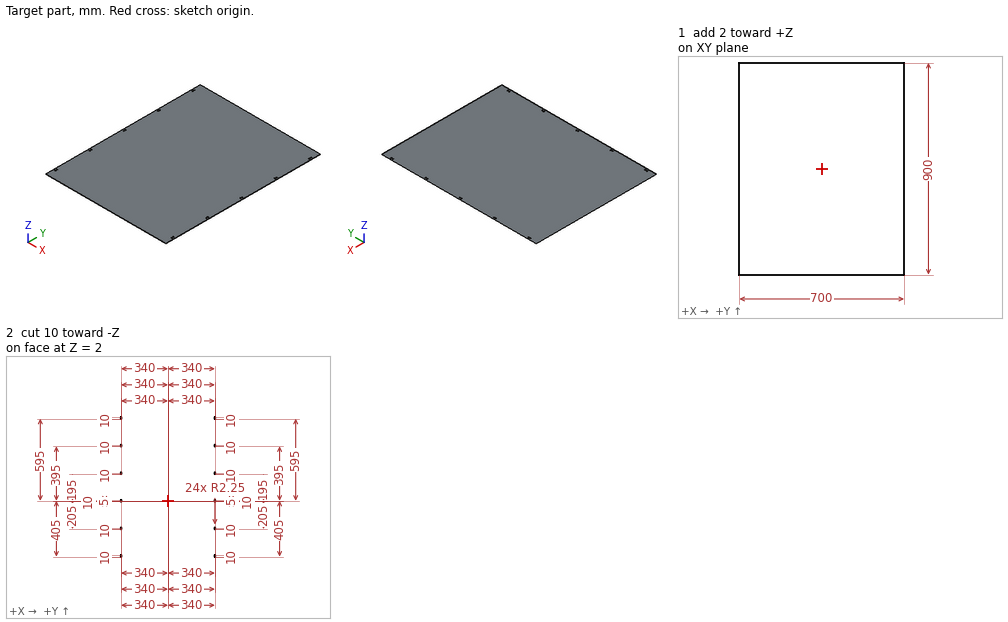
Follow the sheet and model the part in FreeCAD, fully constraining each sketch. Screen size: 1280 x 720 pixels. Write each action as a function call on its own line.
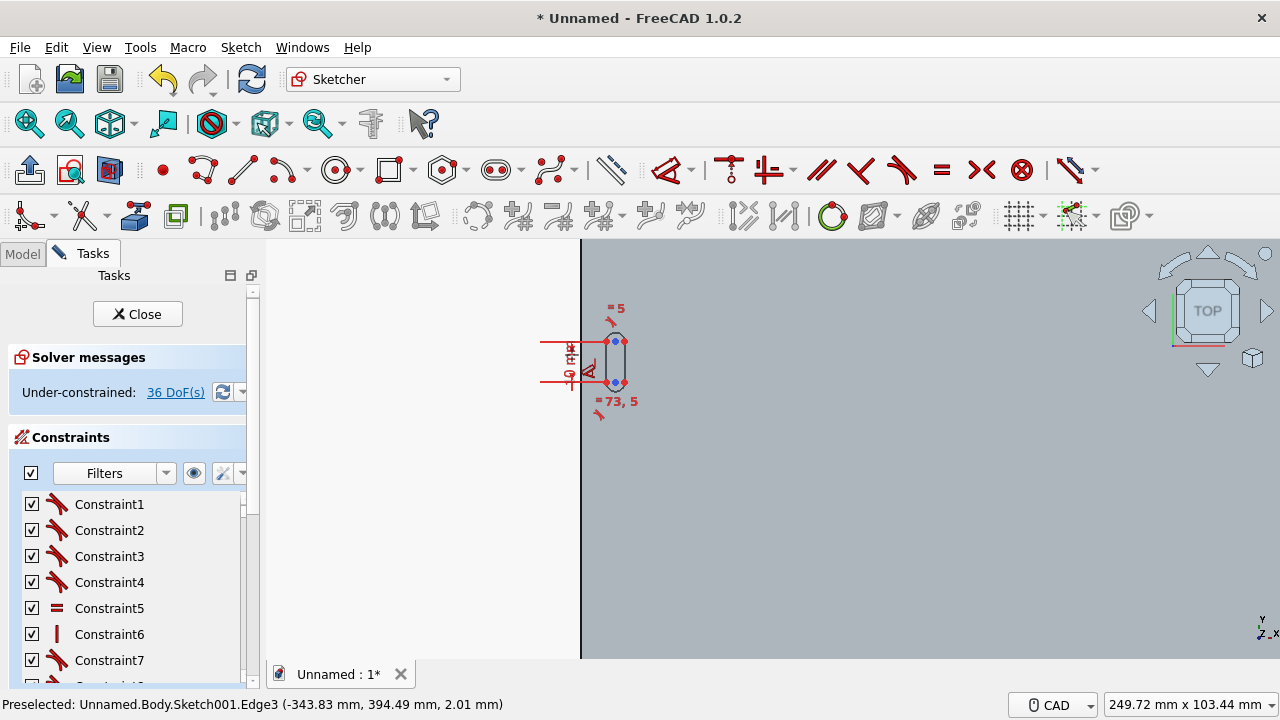
scroll(620, 377, down, 14)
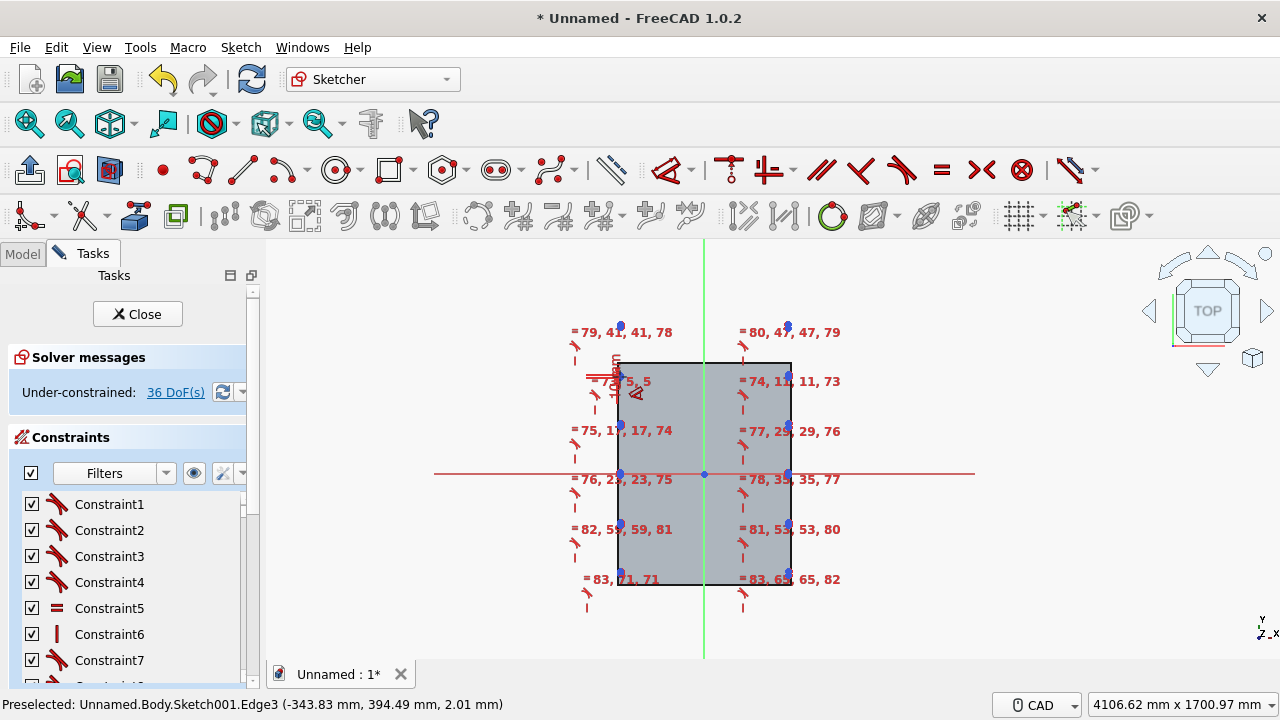
scroll(788, 376, up, 14)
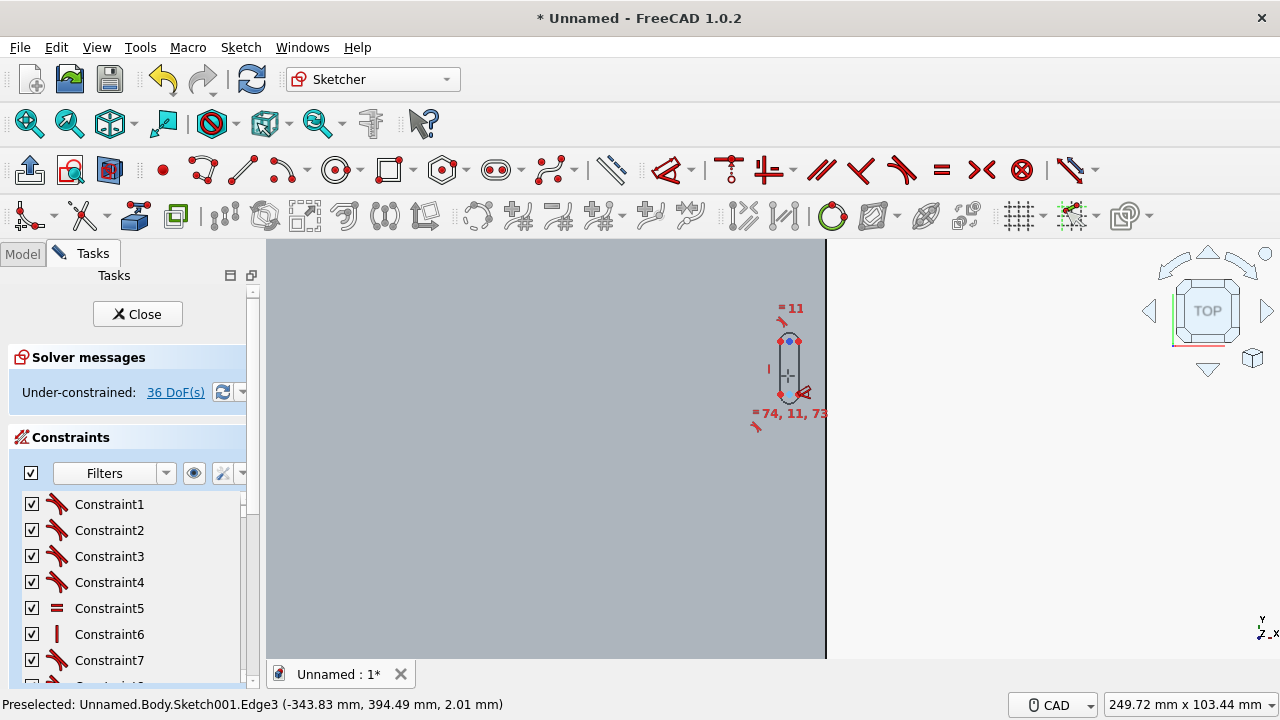
click(780, 379)
click(814, 368)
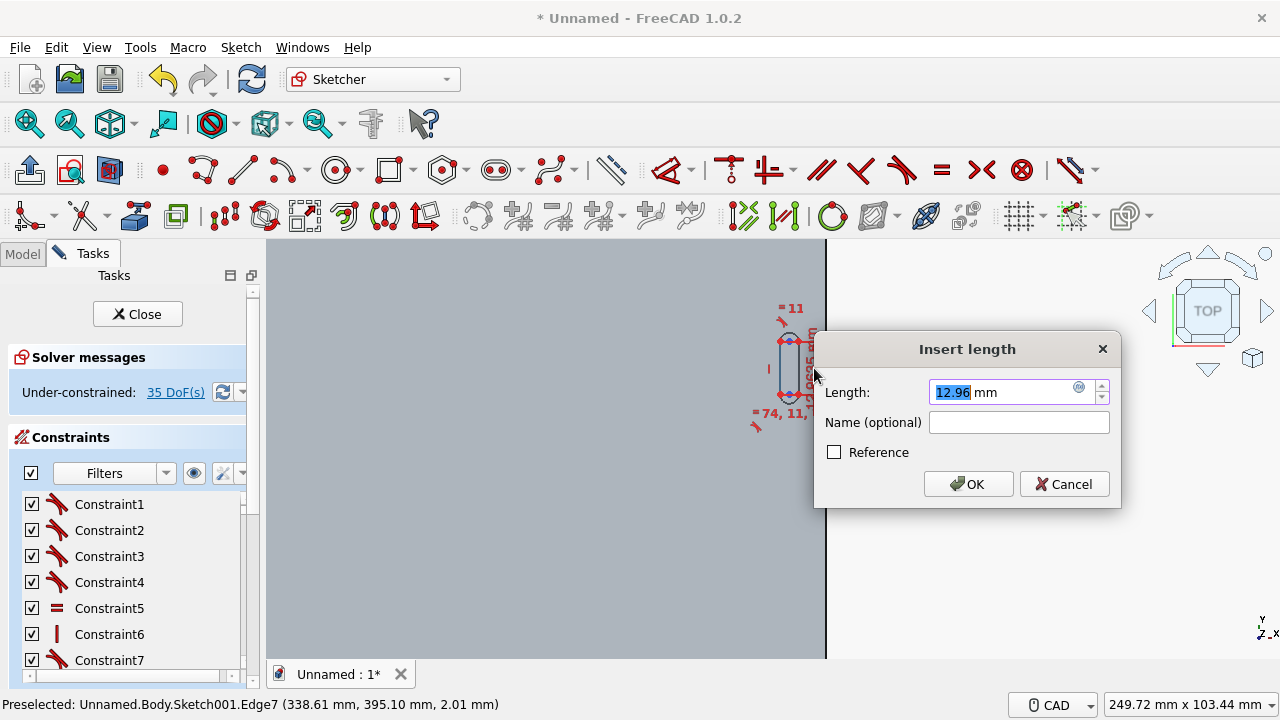
text(10)
key(Return)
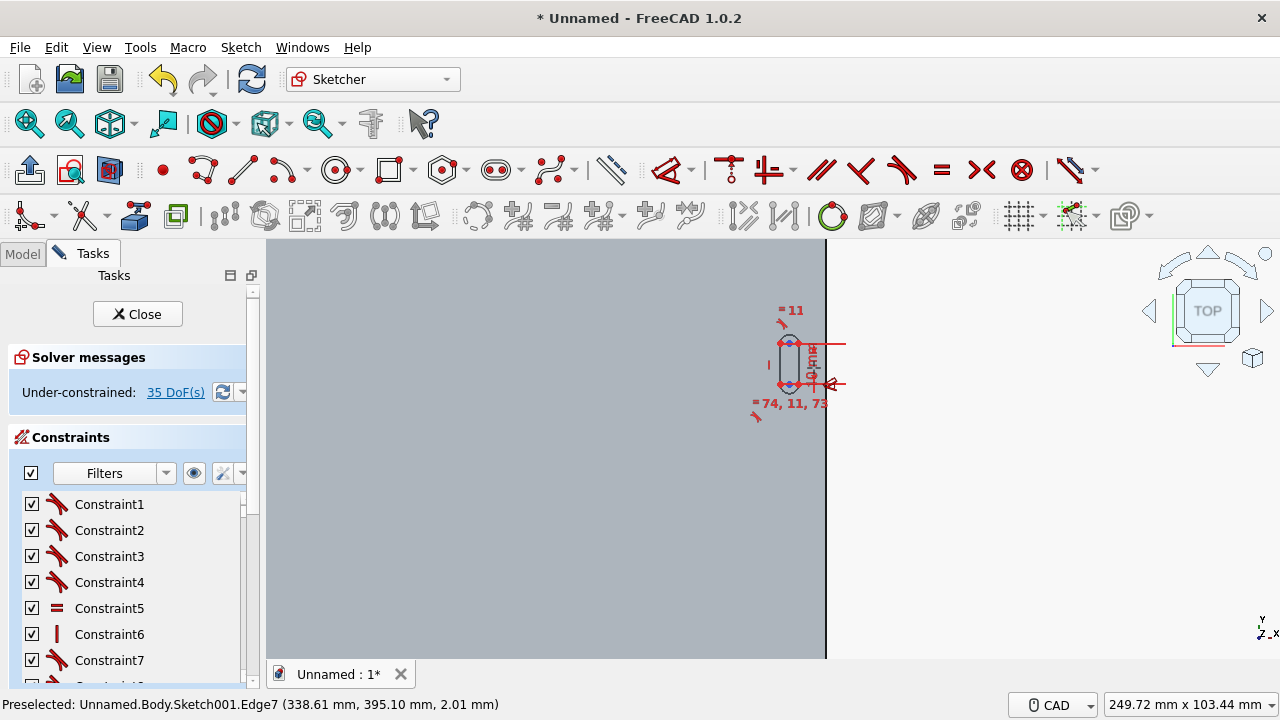
scroll(789, 376, down, 14)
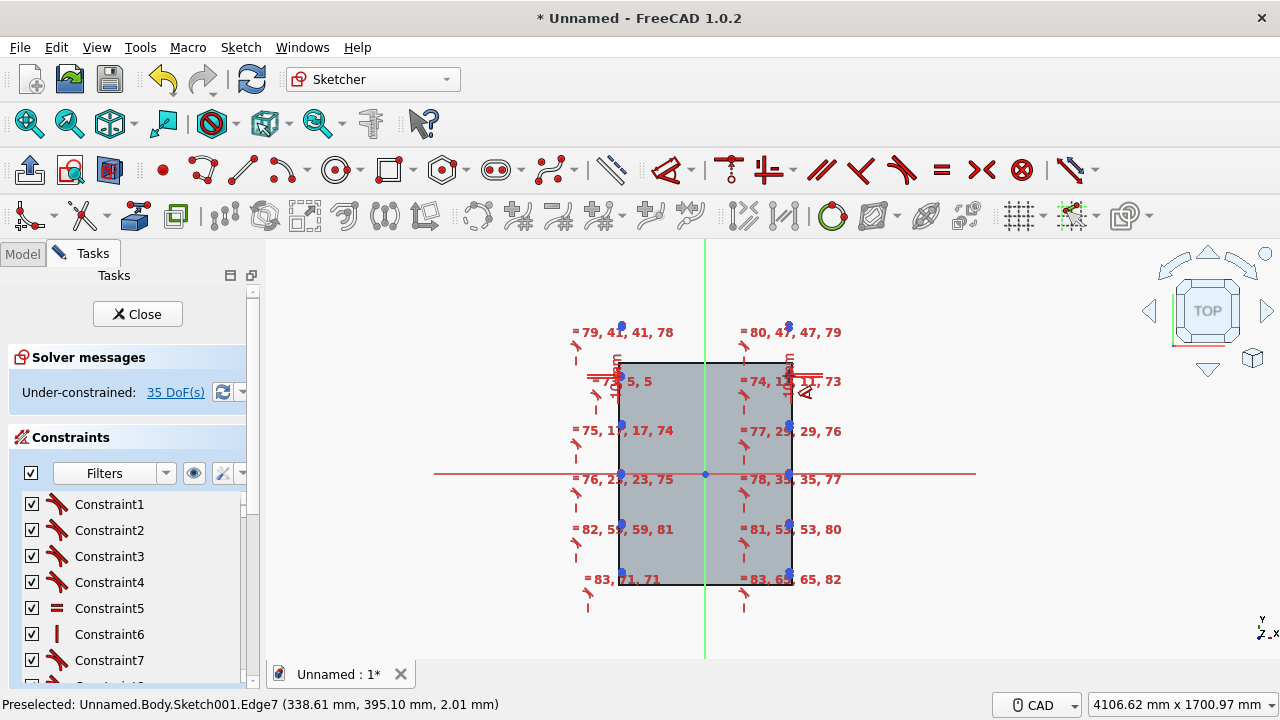
scroll(621, 426, up, 14)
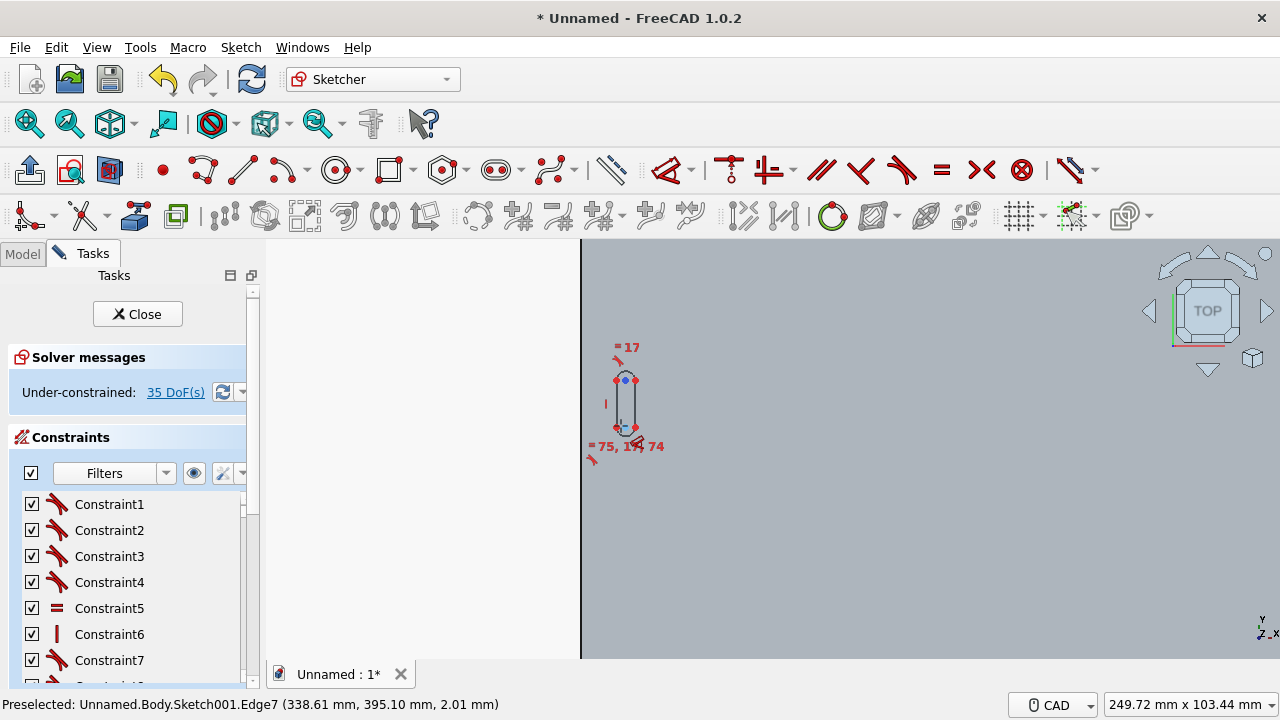
click(617, 413)
click(583, 404)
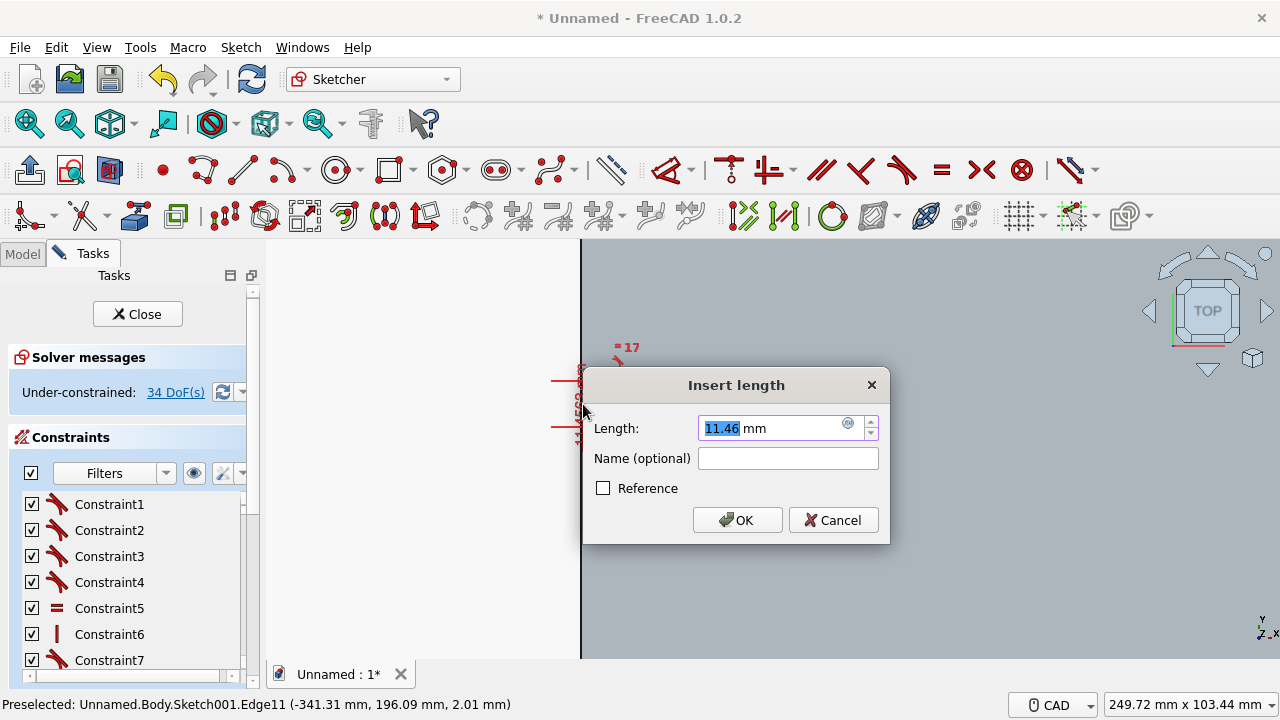
text(10)
key(Return)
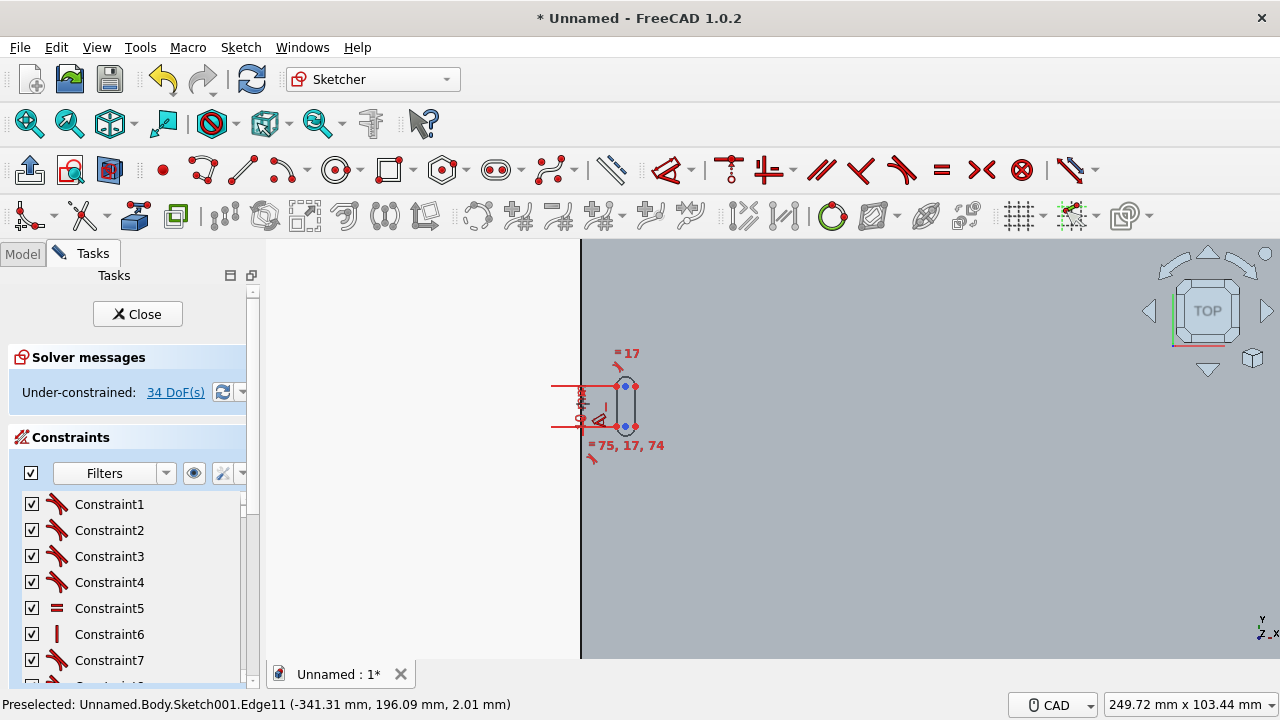
scroll(620, 426, down, 14)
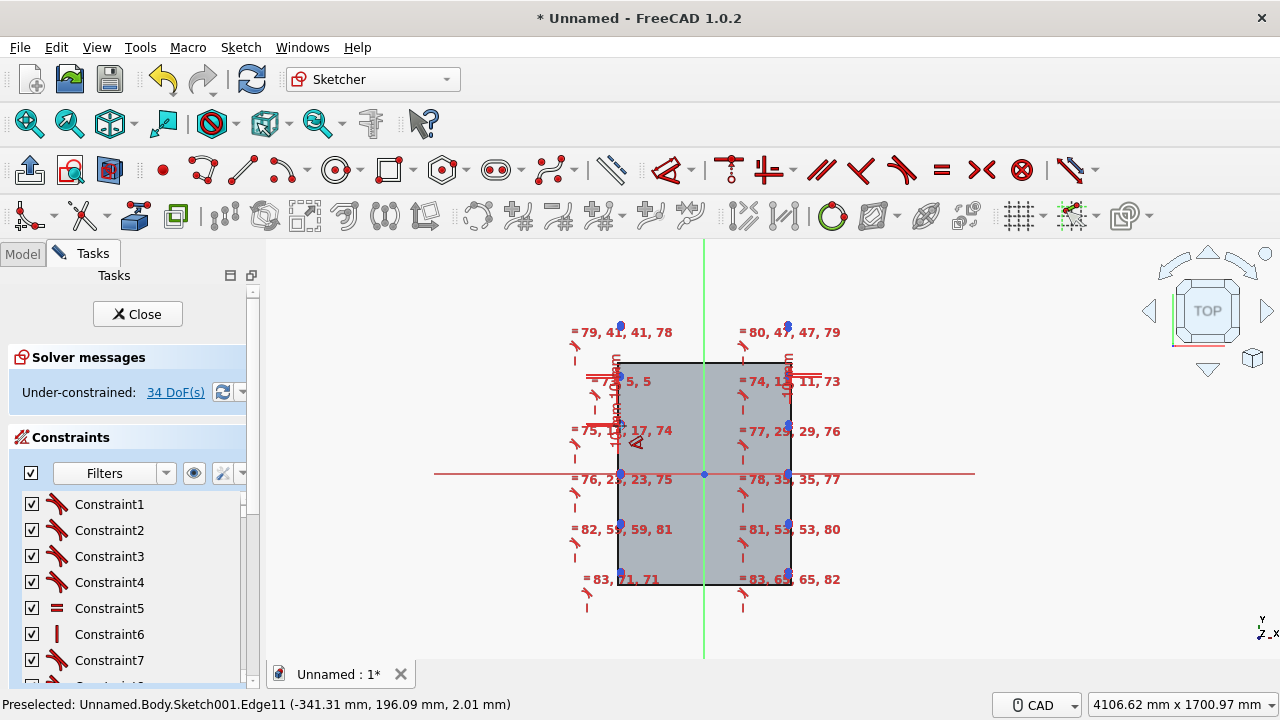
scroll(620, 475, up, 14)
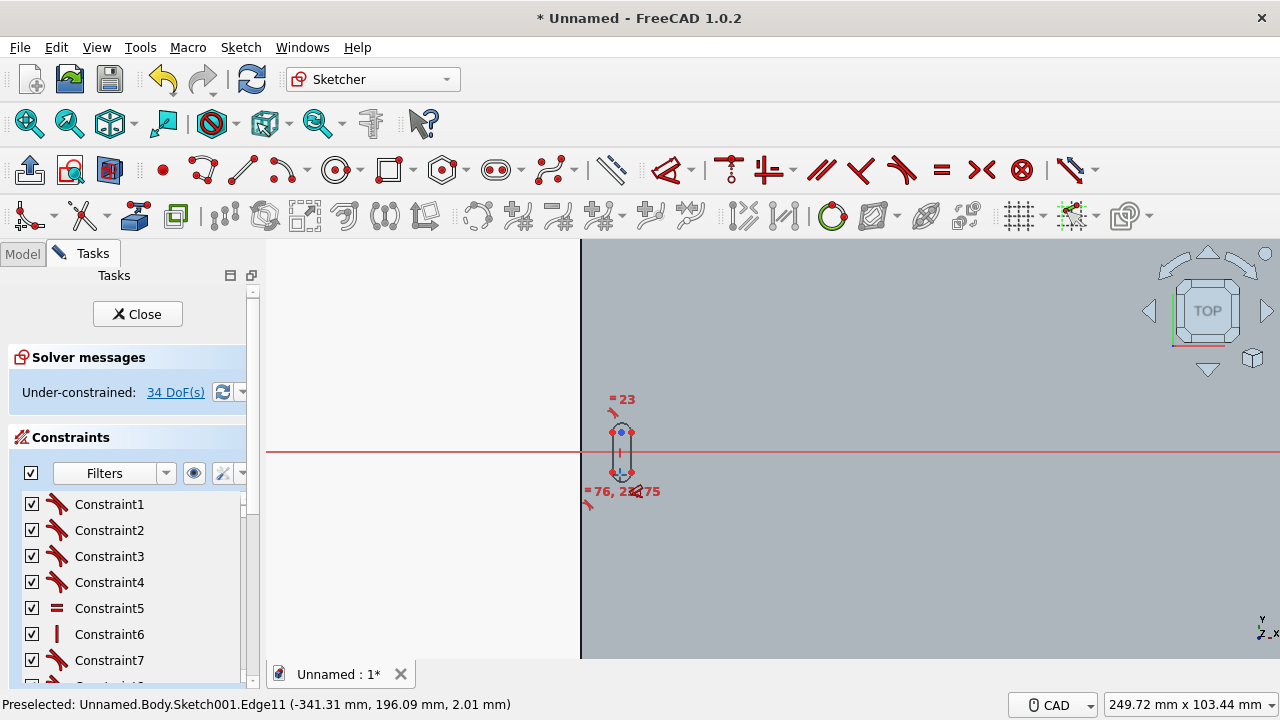
click(613, 461)
click(579, 438)